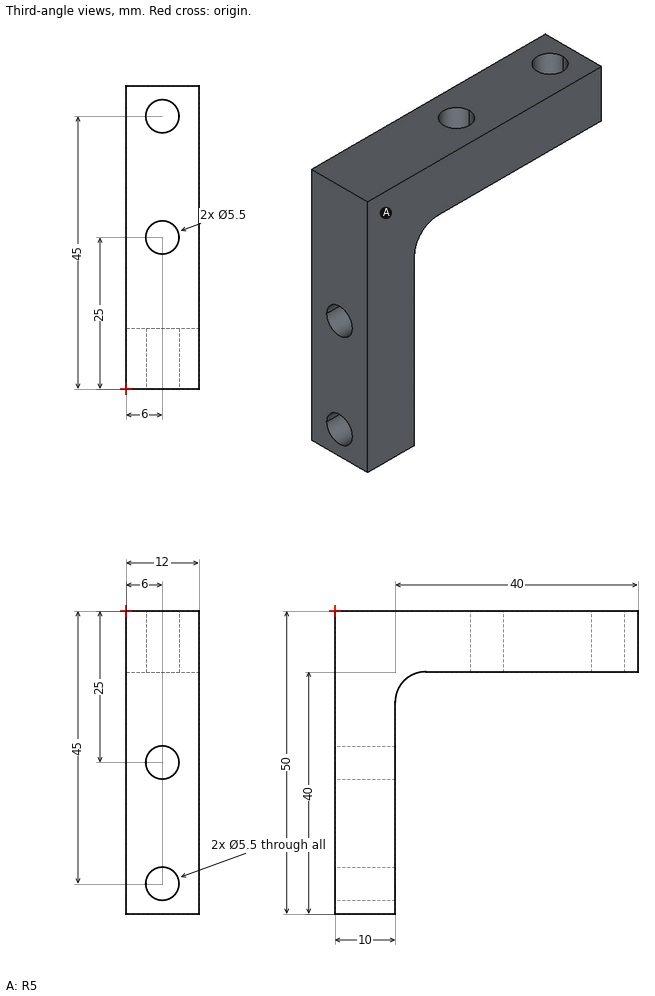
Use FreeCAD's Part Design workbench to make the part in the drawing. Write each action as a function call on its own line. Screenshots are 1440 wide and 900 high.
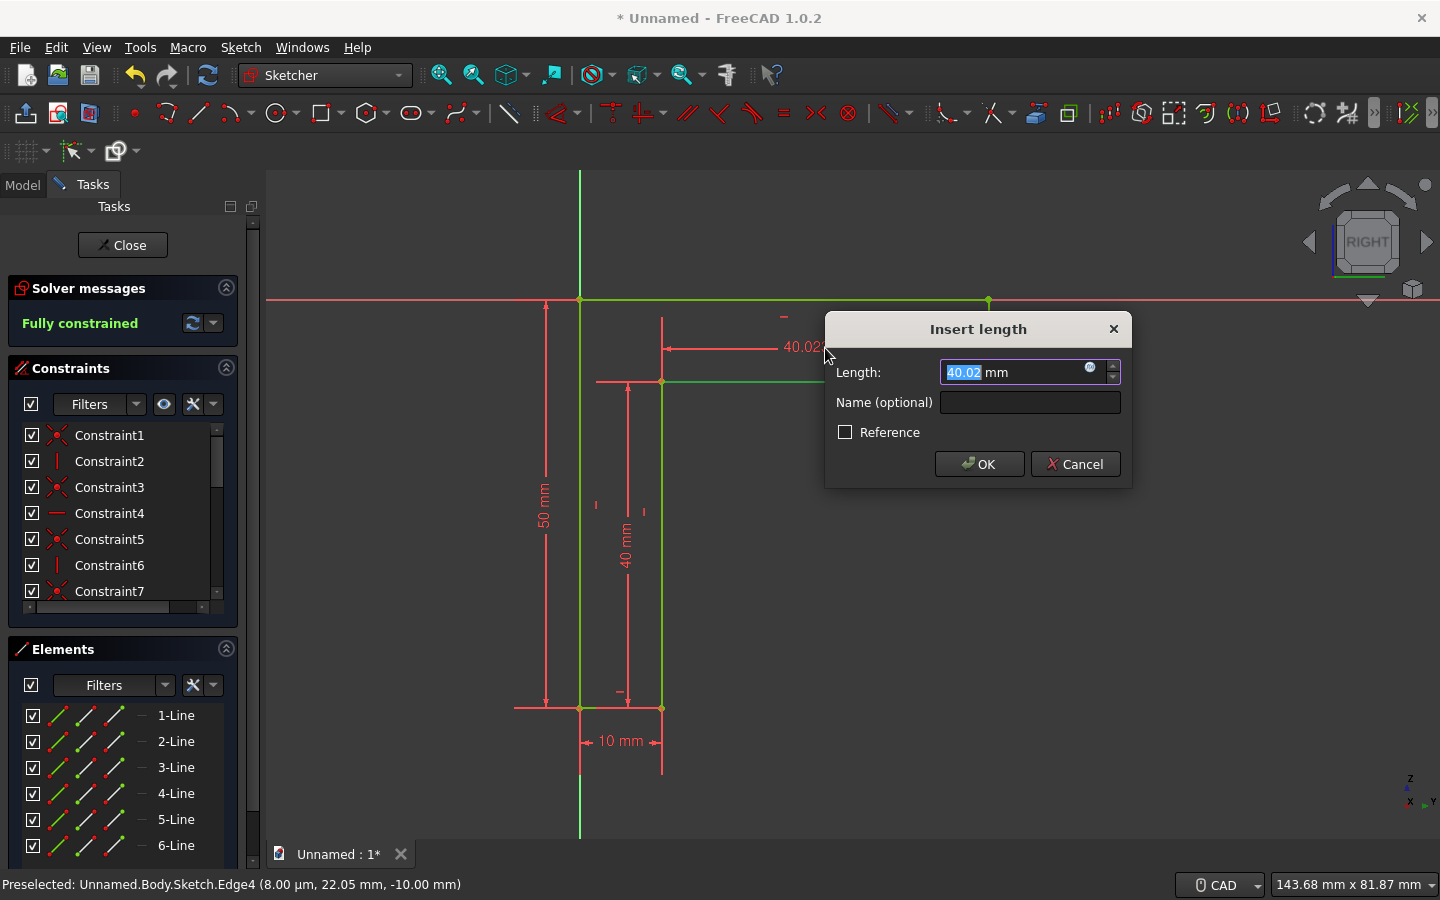
text(40)
key(Return)
key(Escape)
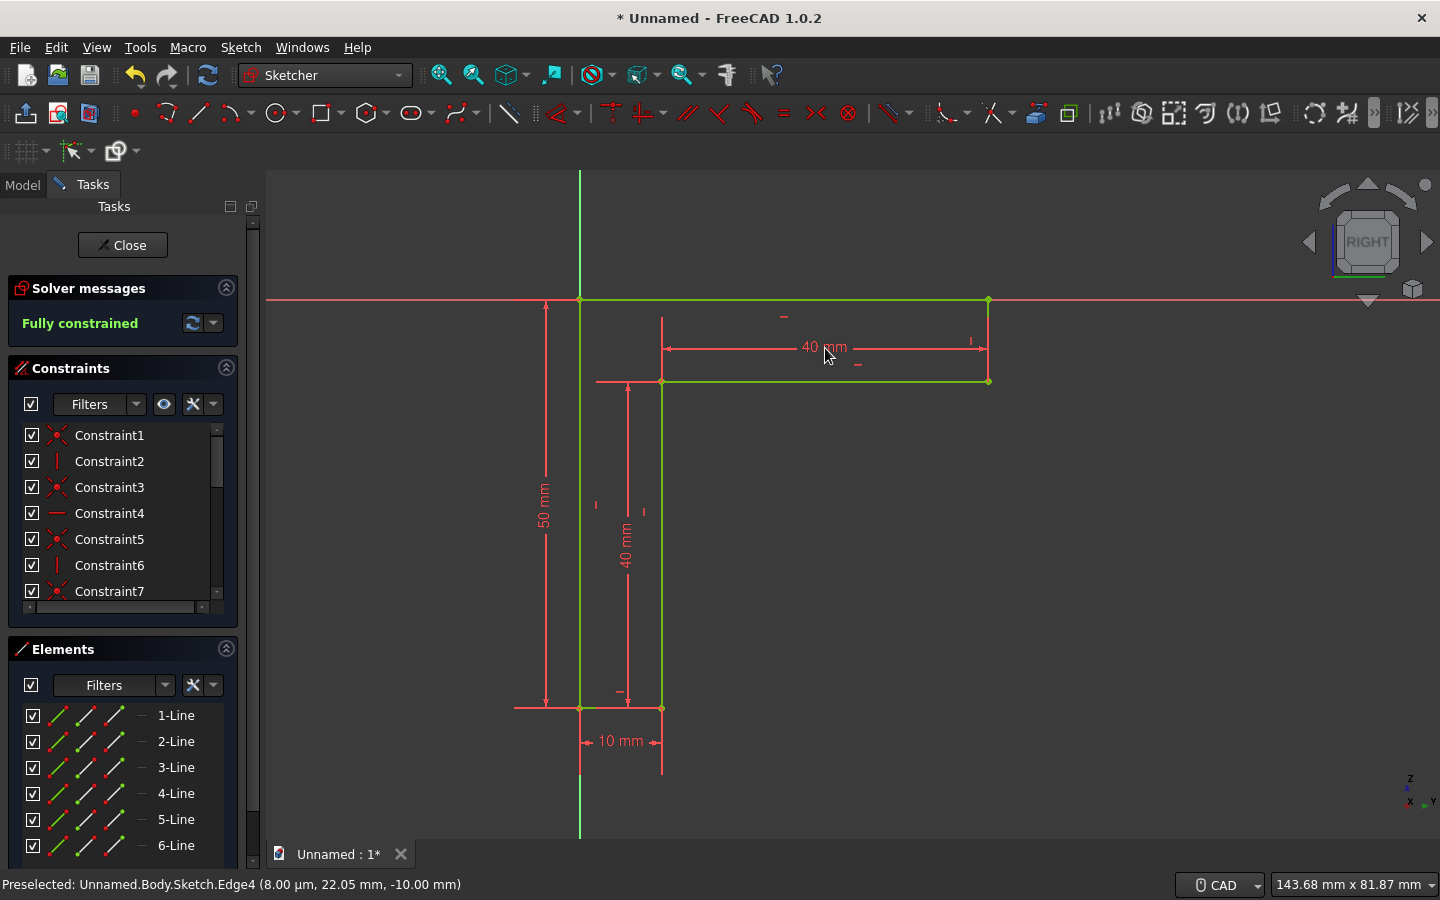
click(123, 245)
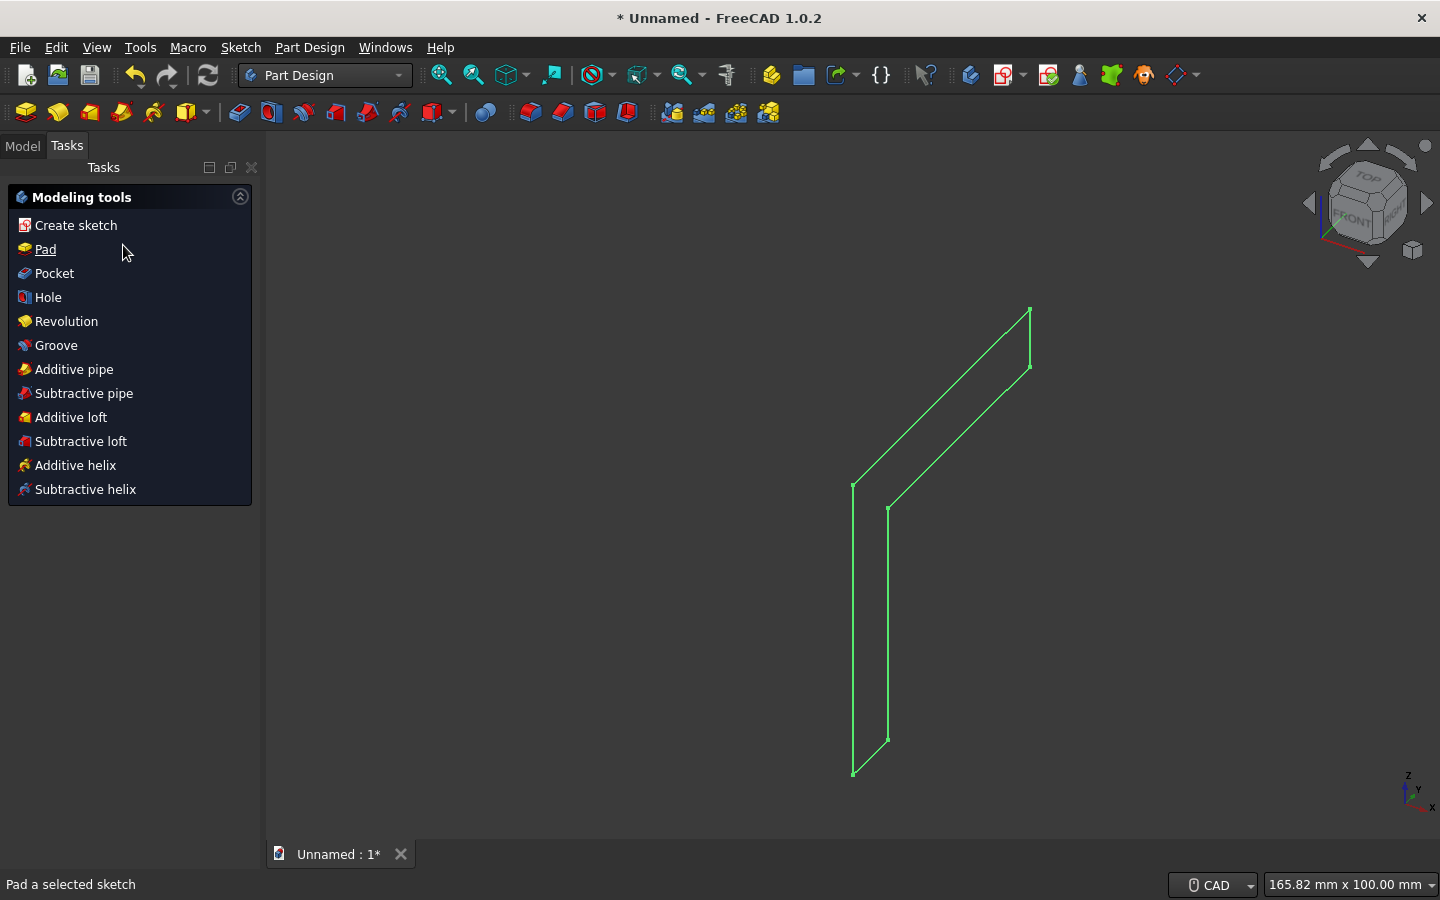
click(26, 112)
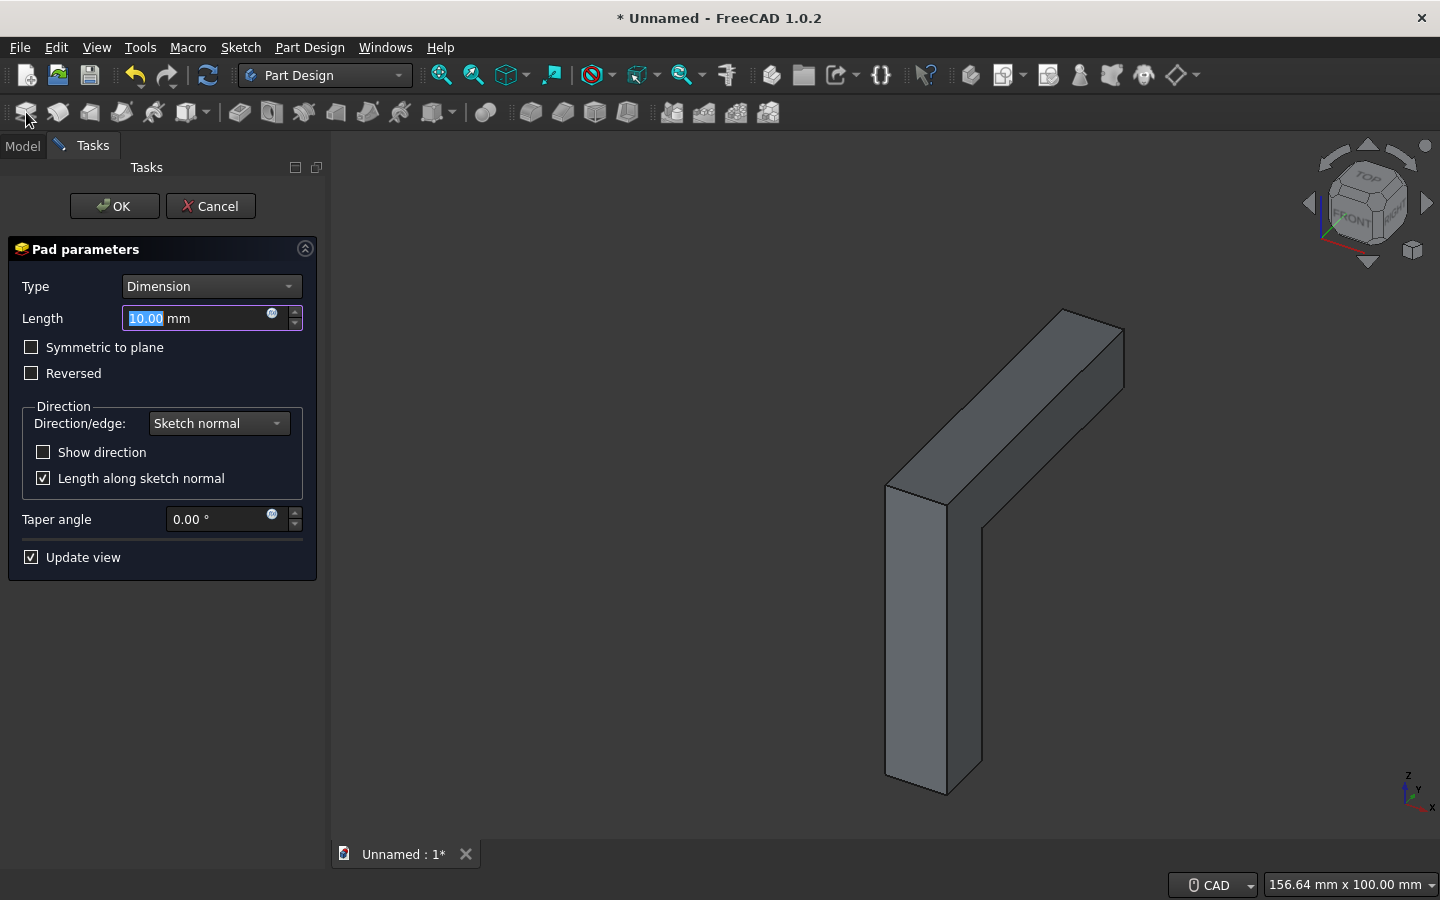
text(12)
key(Tab)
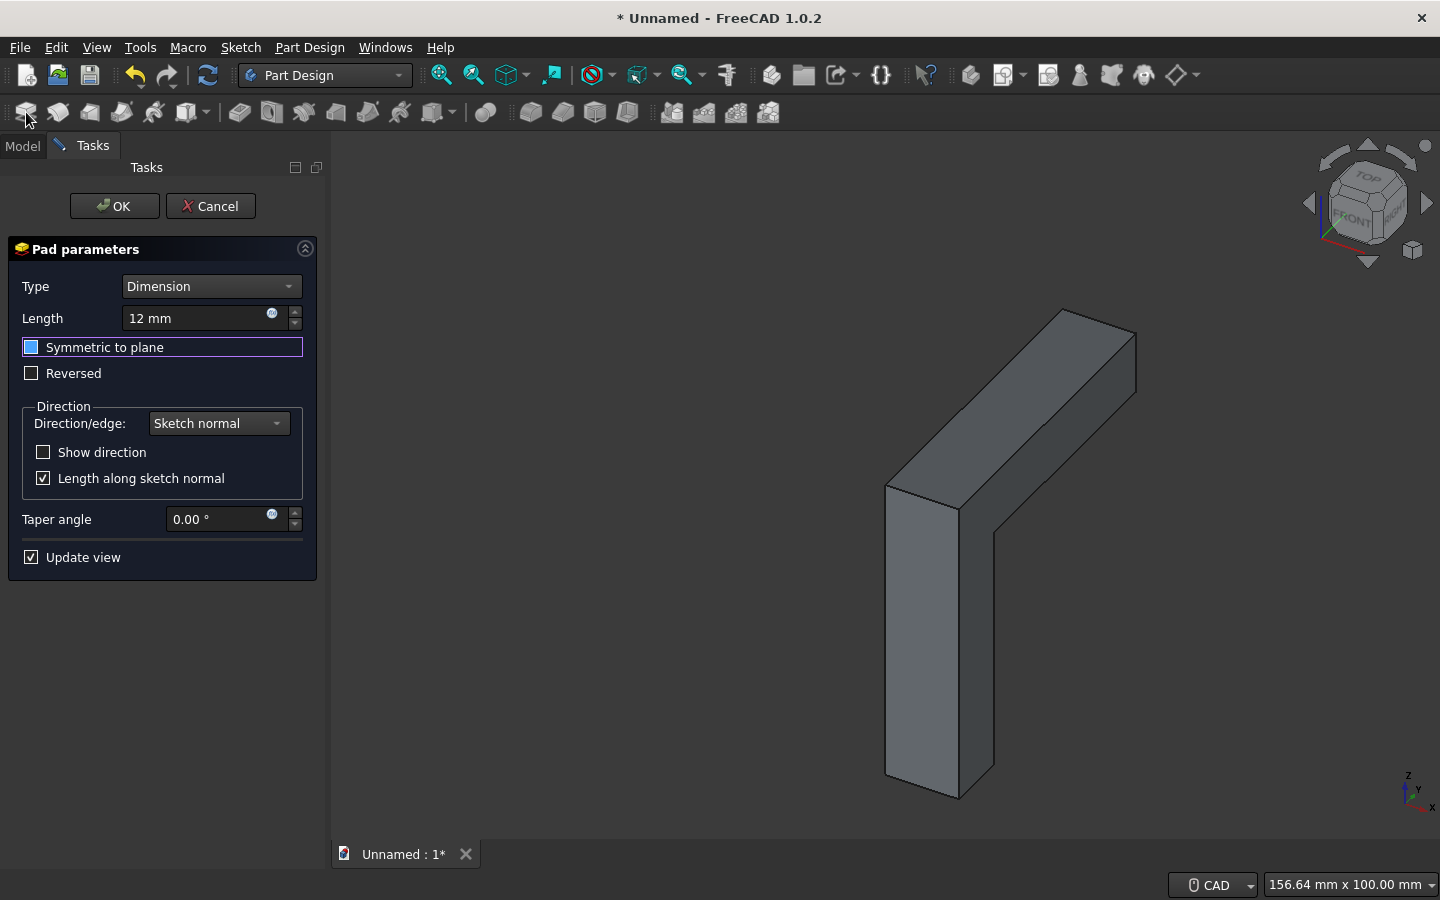
click(115, 206)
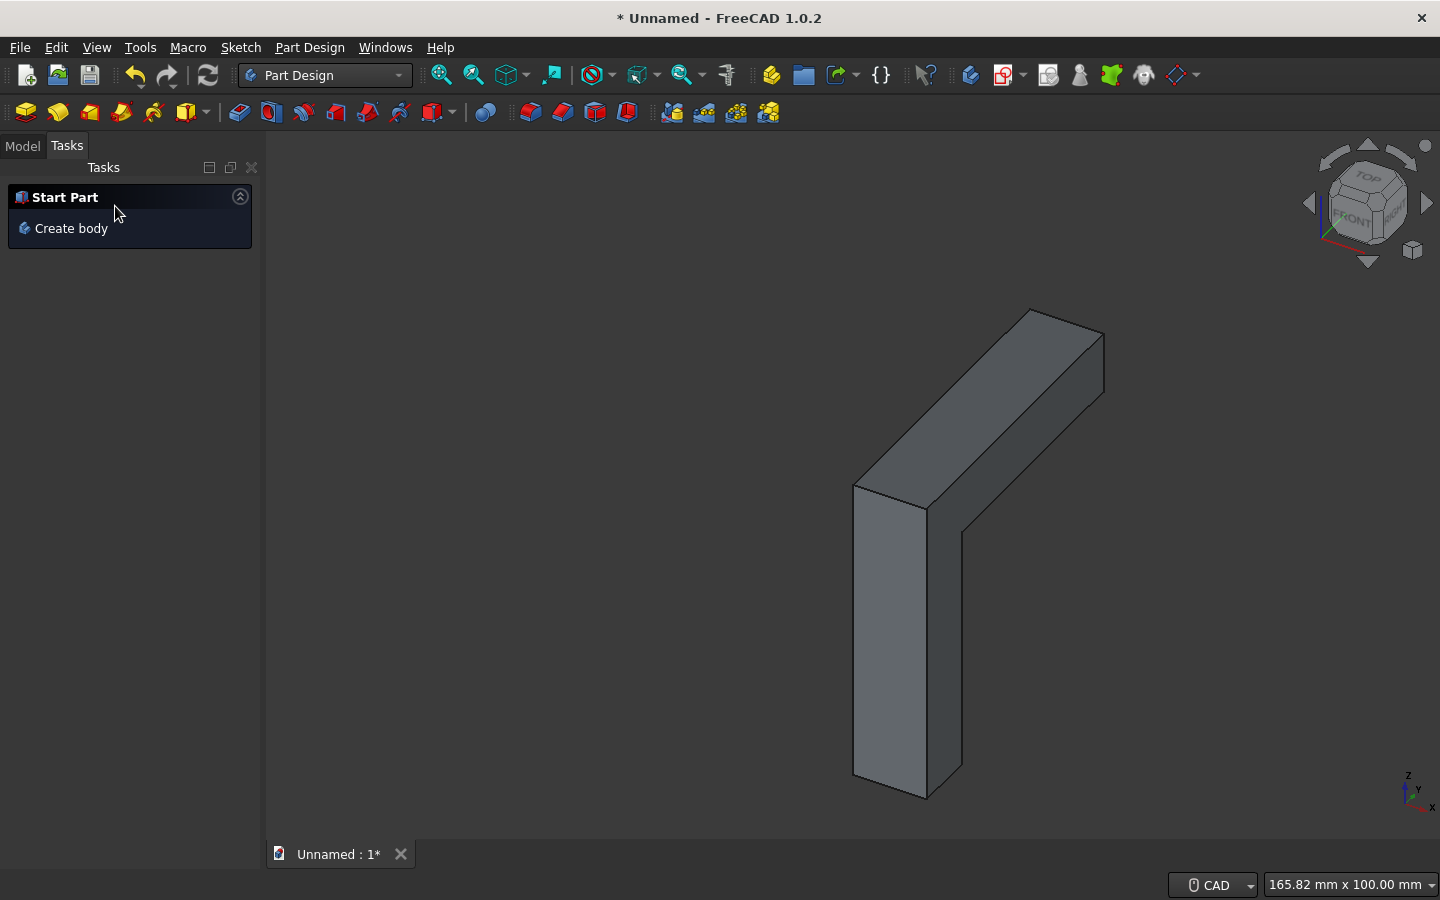
key(0)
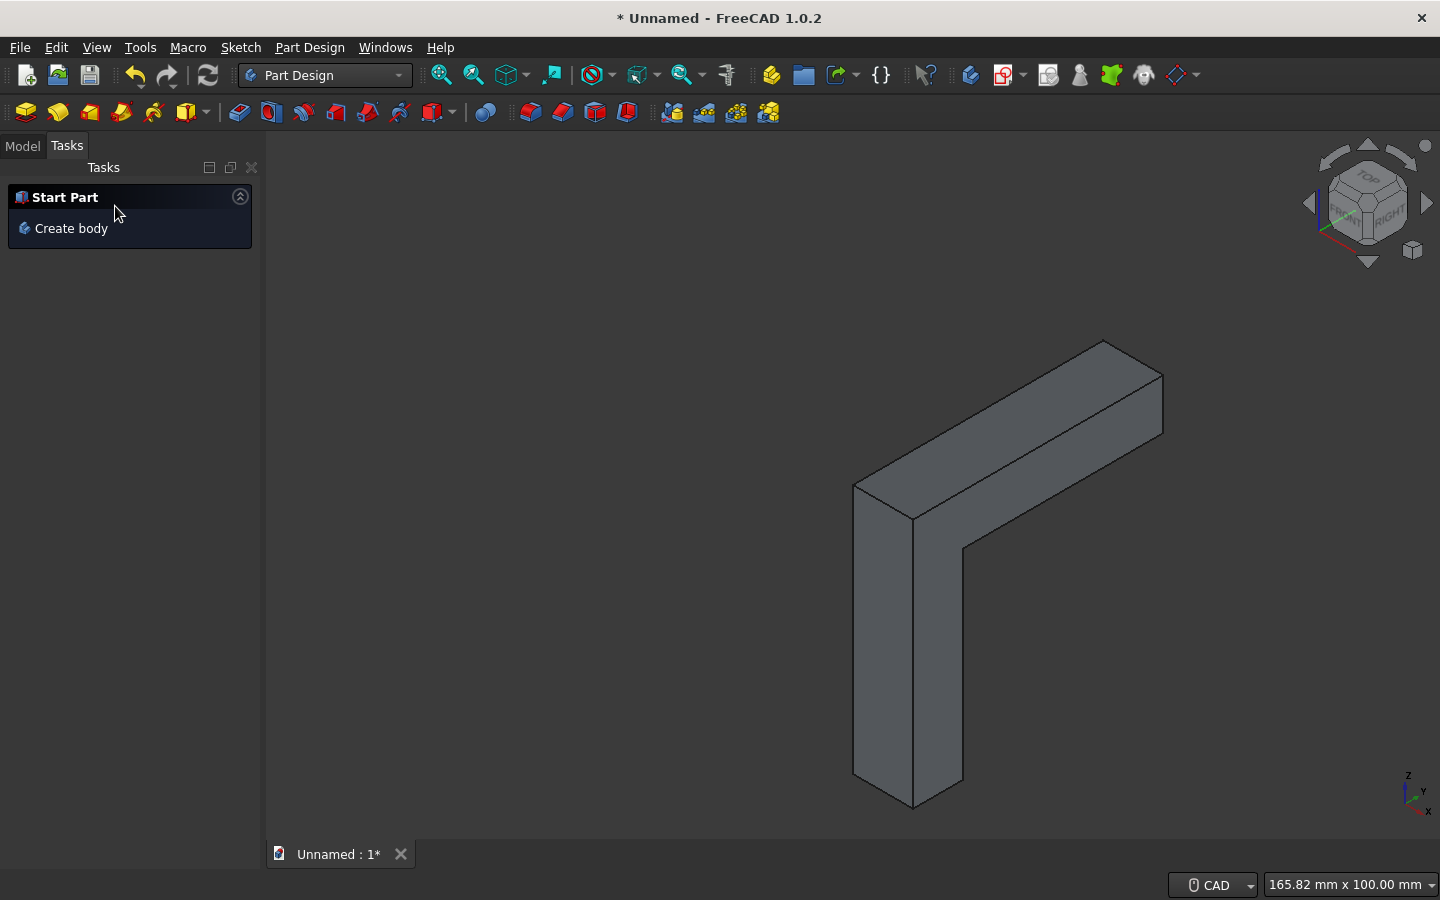
key(2)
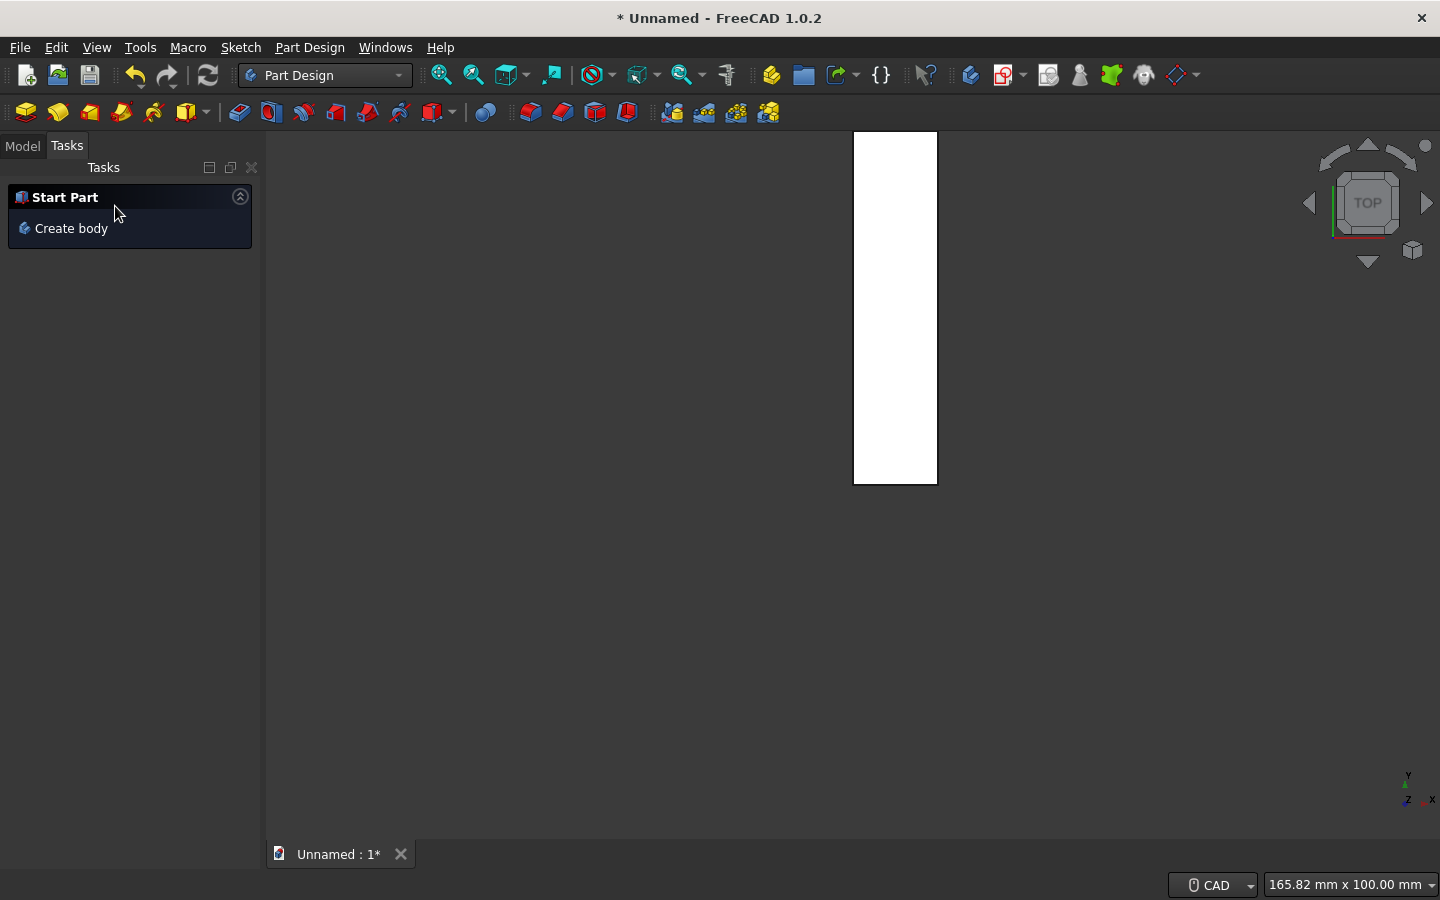
click(442, 76)